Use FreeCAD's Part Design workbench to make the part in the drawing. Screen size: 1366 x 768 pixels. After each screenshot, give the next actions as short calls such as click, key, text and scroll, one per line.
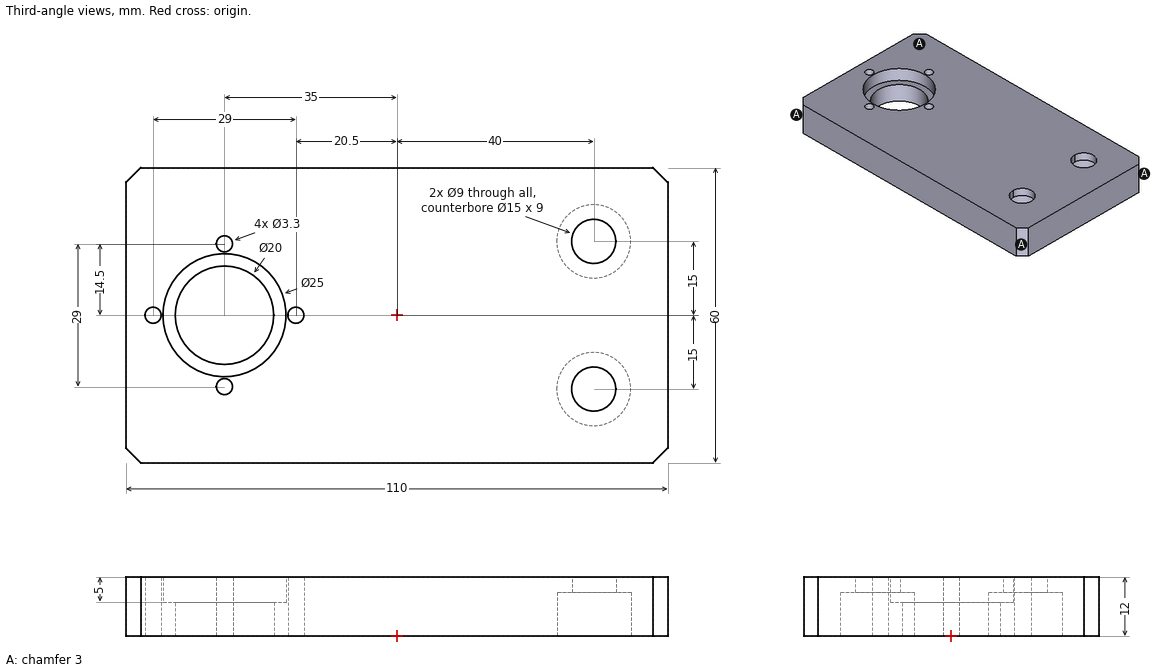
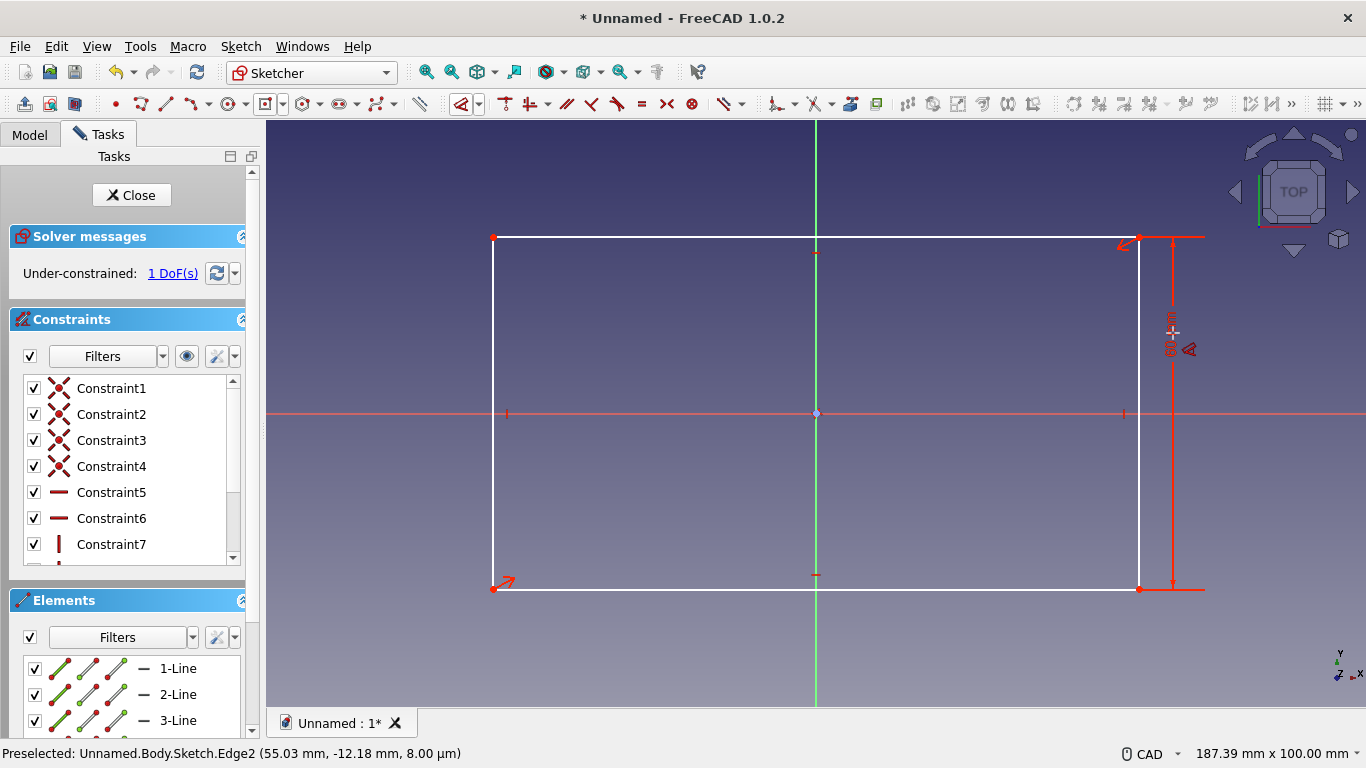
click(687, 590)
click(667, 624)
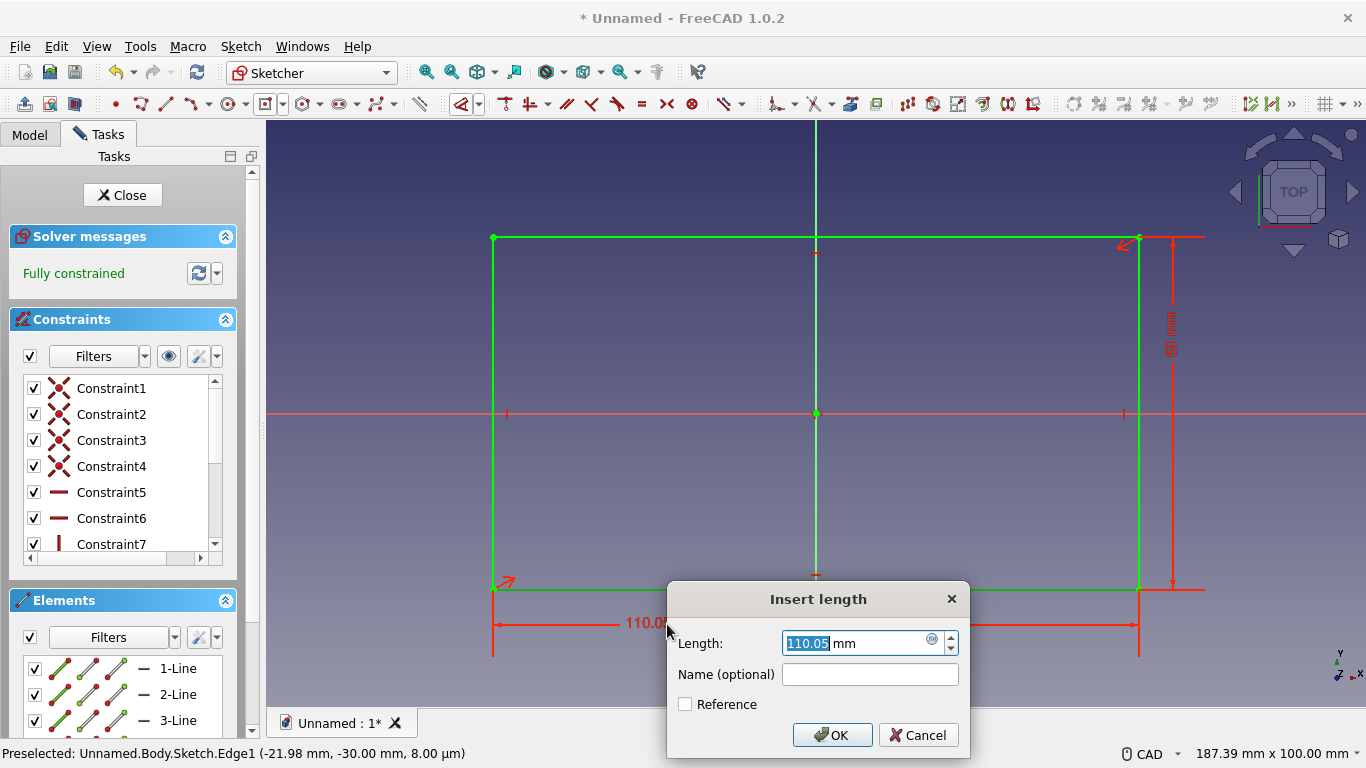
text(110)
key(Return)
key(Escape)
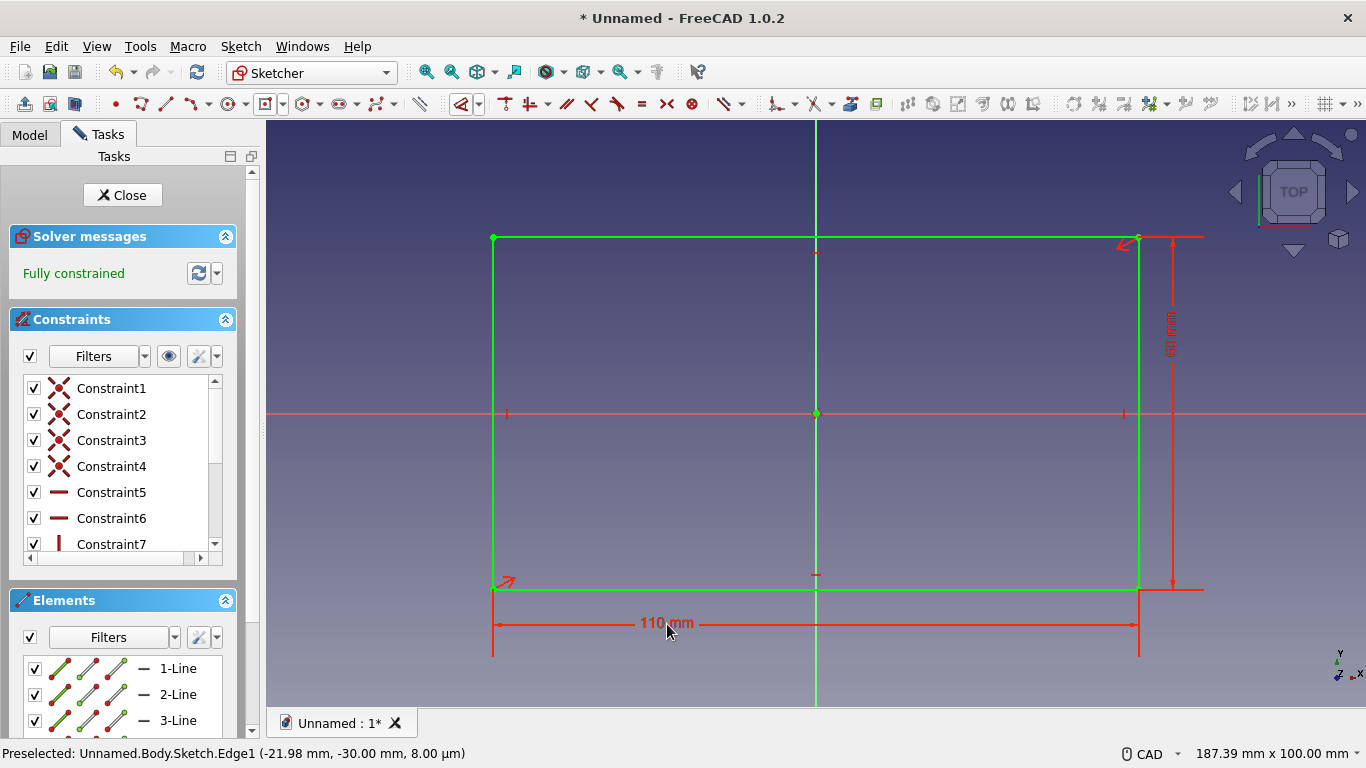
click(123, 195)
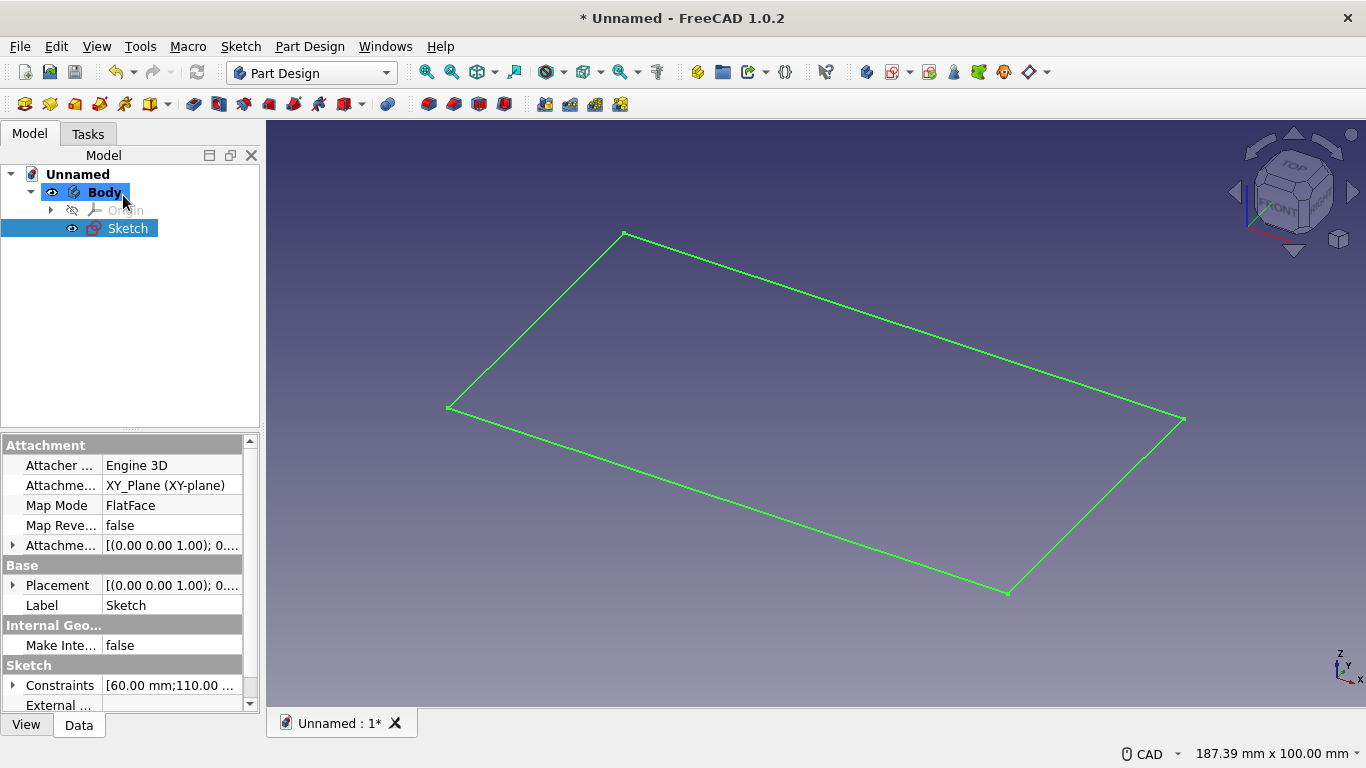
click(25, 104)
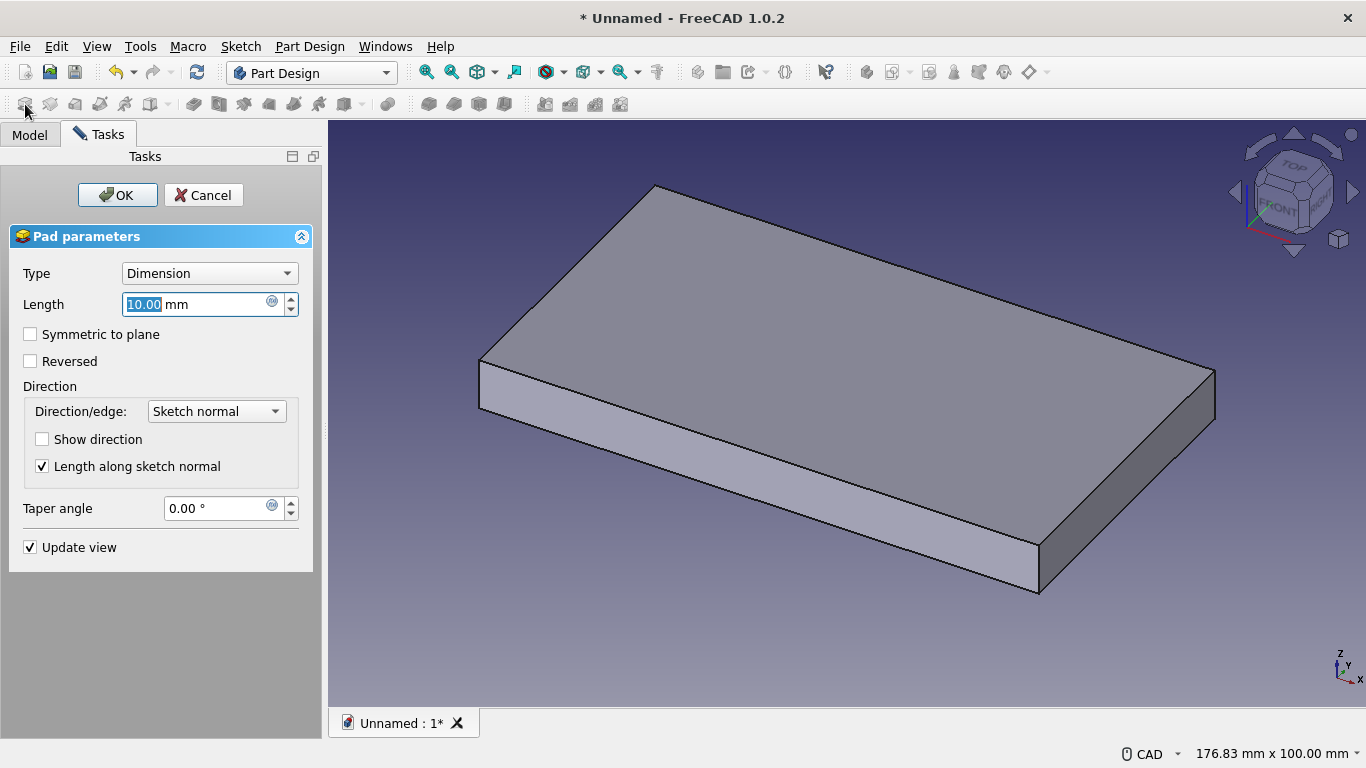
text(12)
key(Tab)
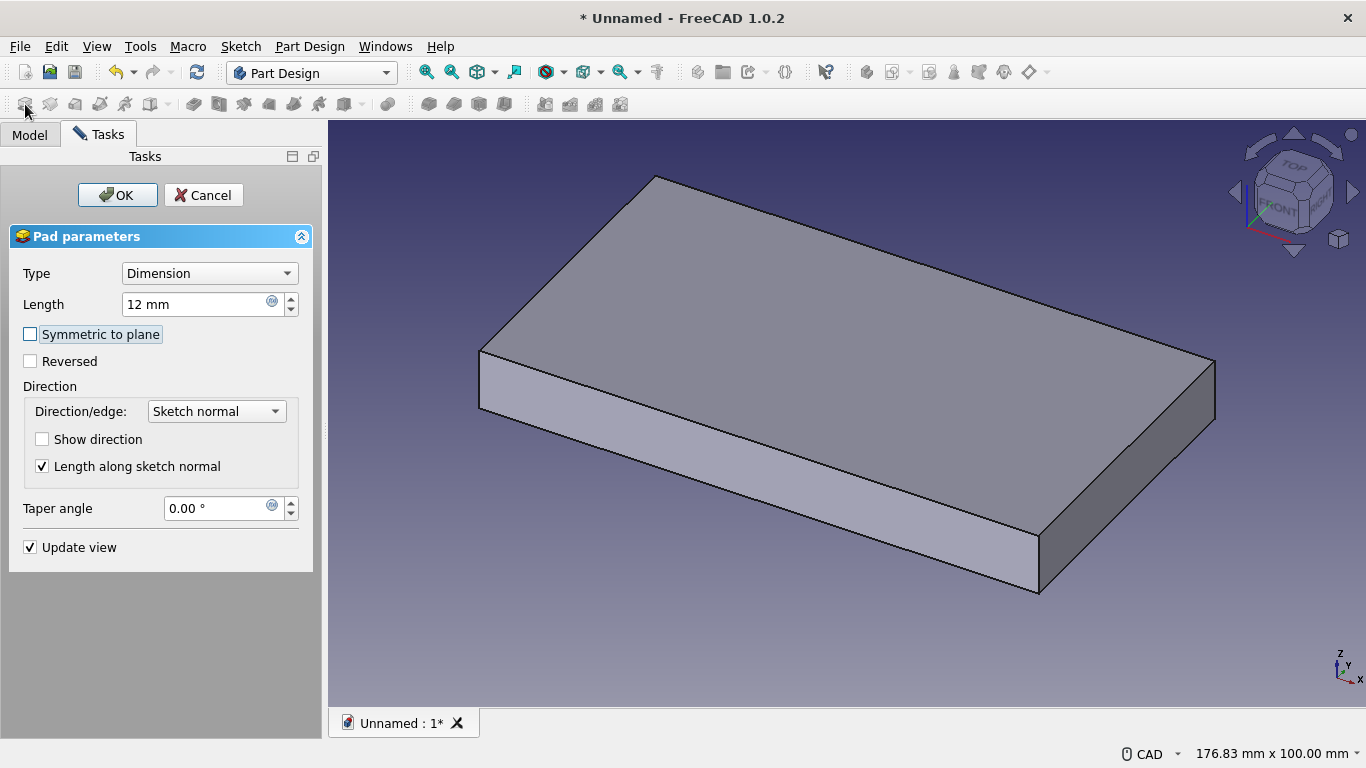
click(118, 195)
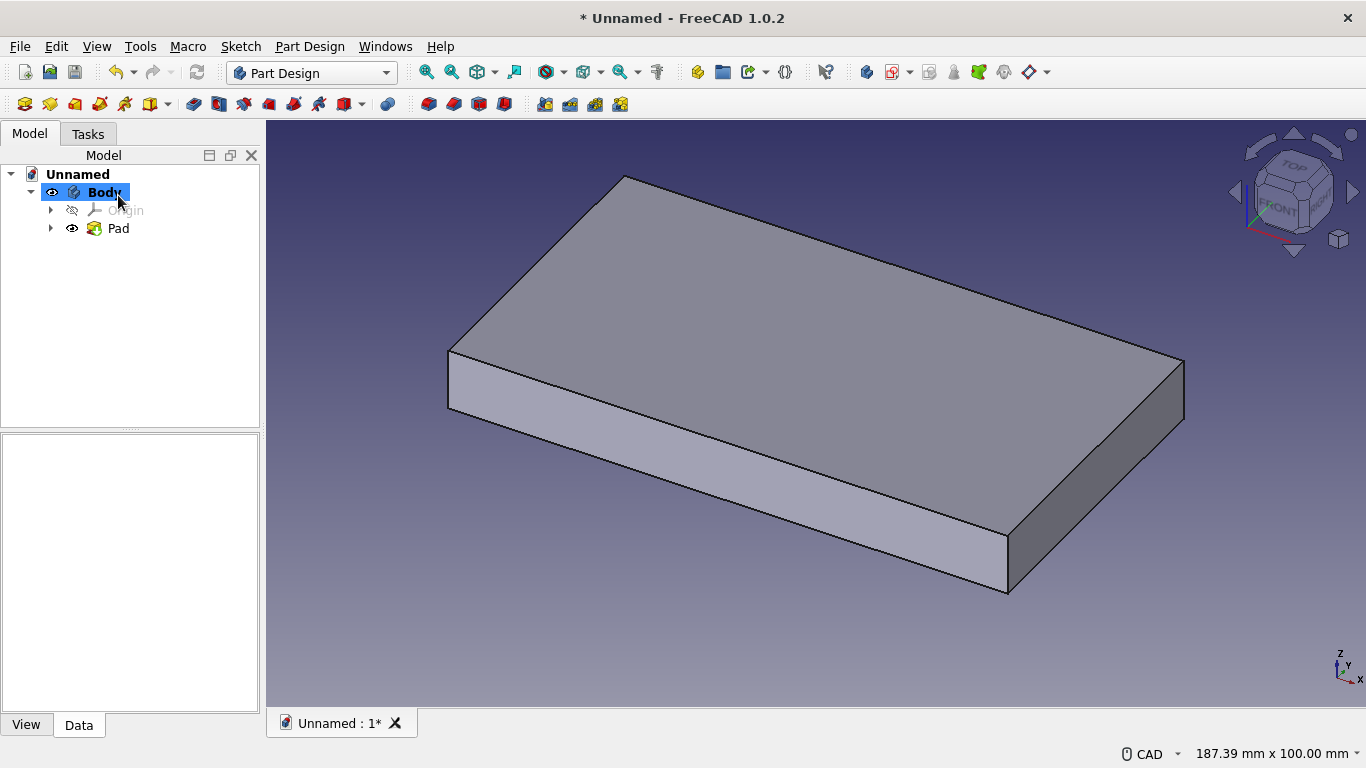
click(896, 381)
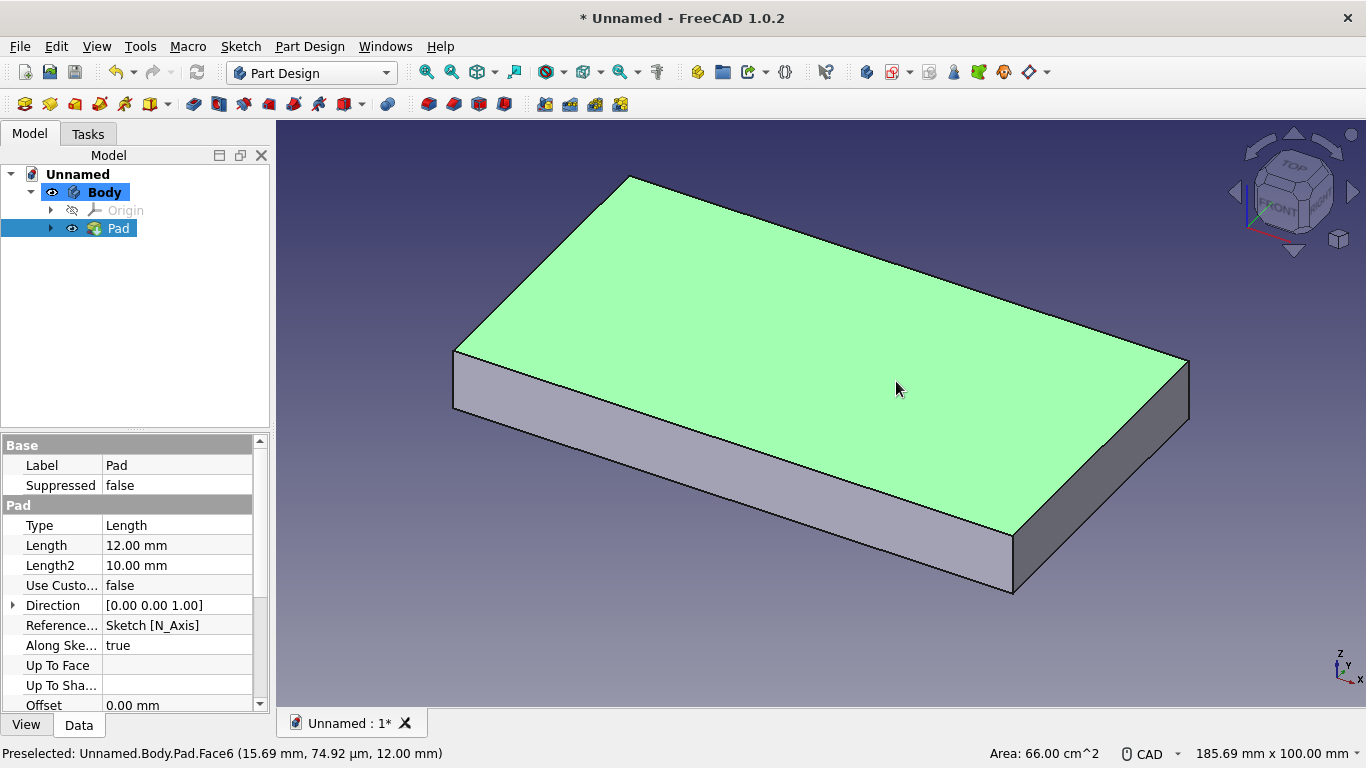
click(892, 72)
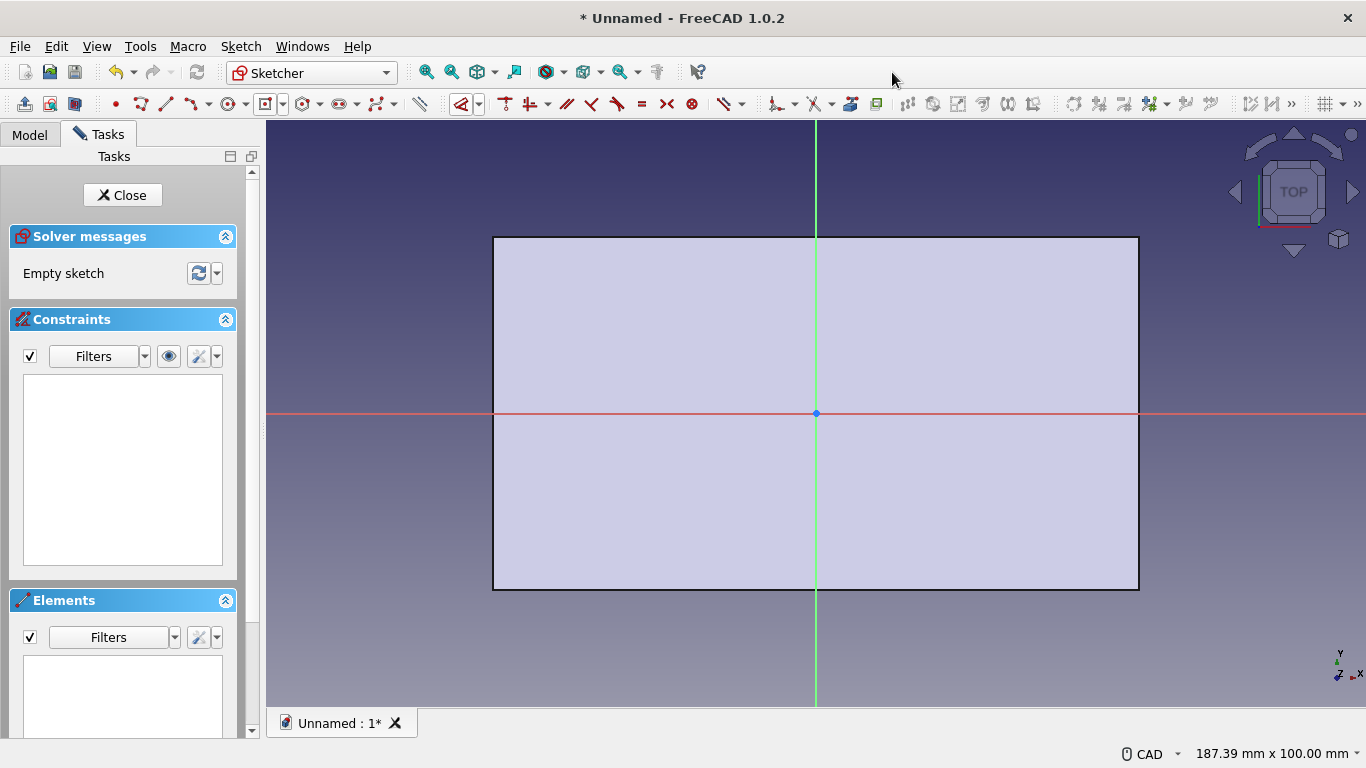
scroll(619, 413, up, 4)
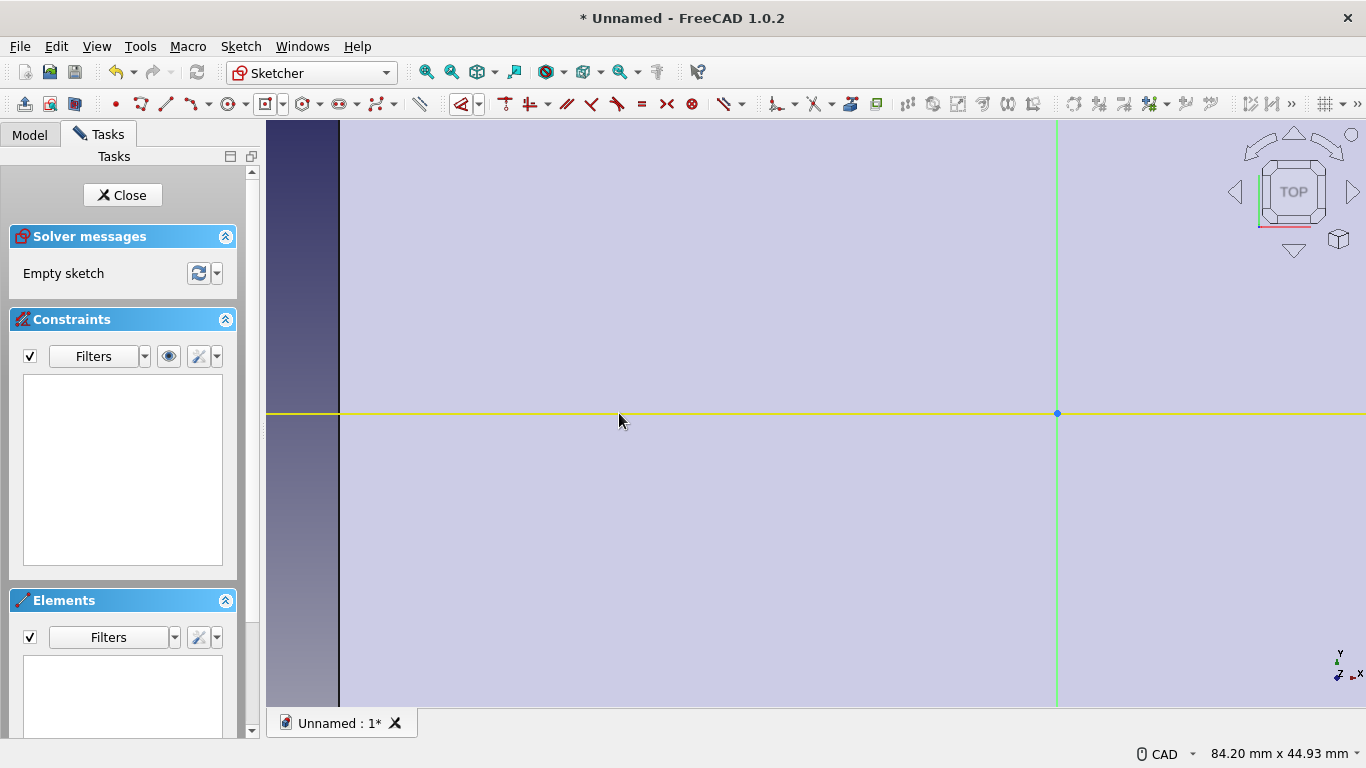
click(228, 104)